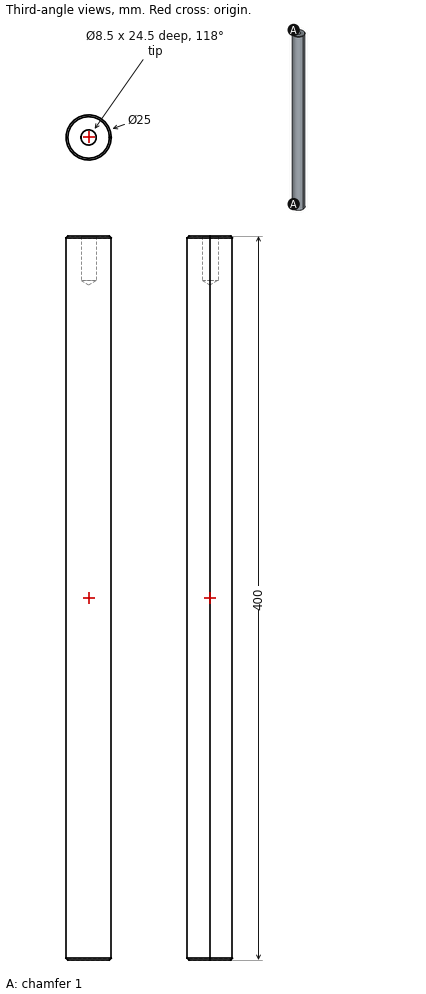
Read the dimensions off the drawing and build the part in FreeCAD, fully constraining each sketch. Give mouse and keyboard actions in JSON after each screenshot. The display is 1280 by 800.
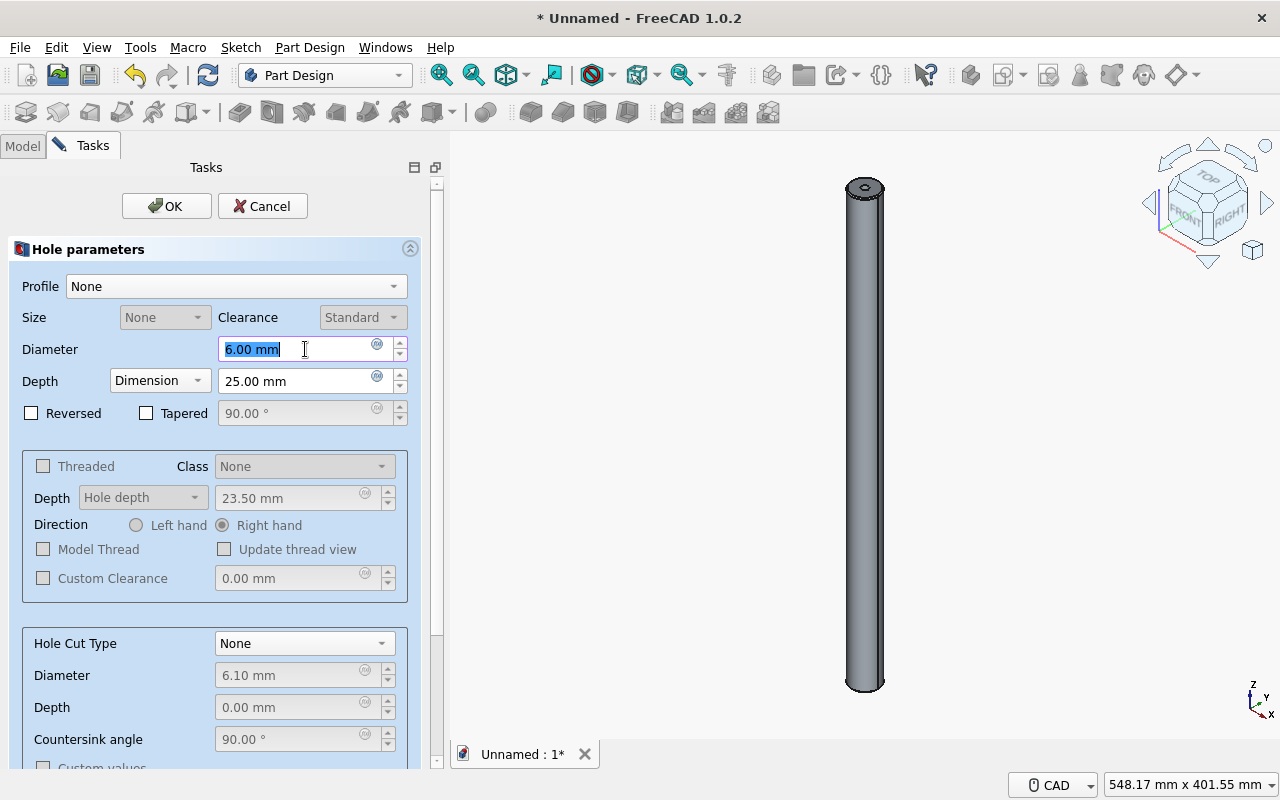
{"action": "type", "text": "8.5"}
{"action": "key", "text": "Tab"}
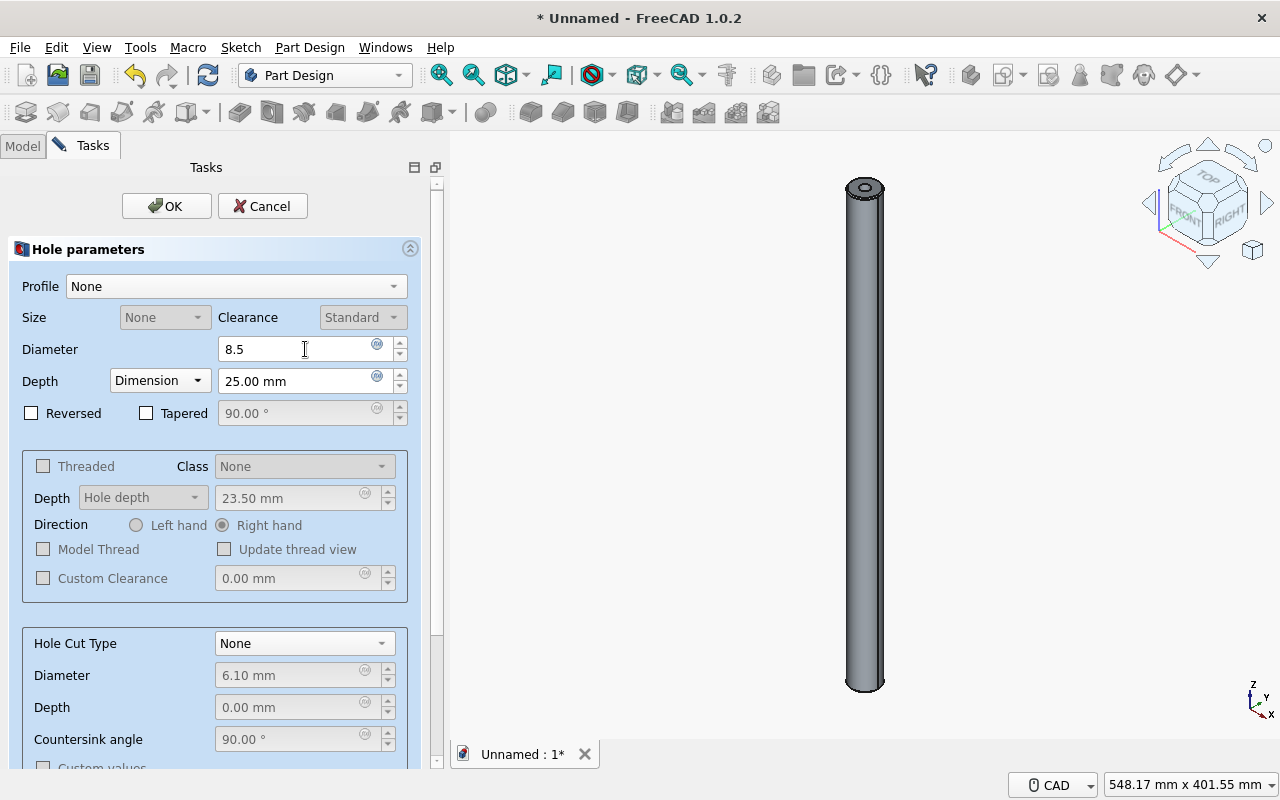
{"action": "triple_click", "coordinate": [305, 381]}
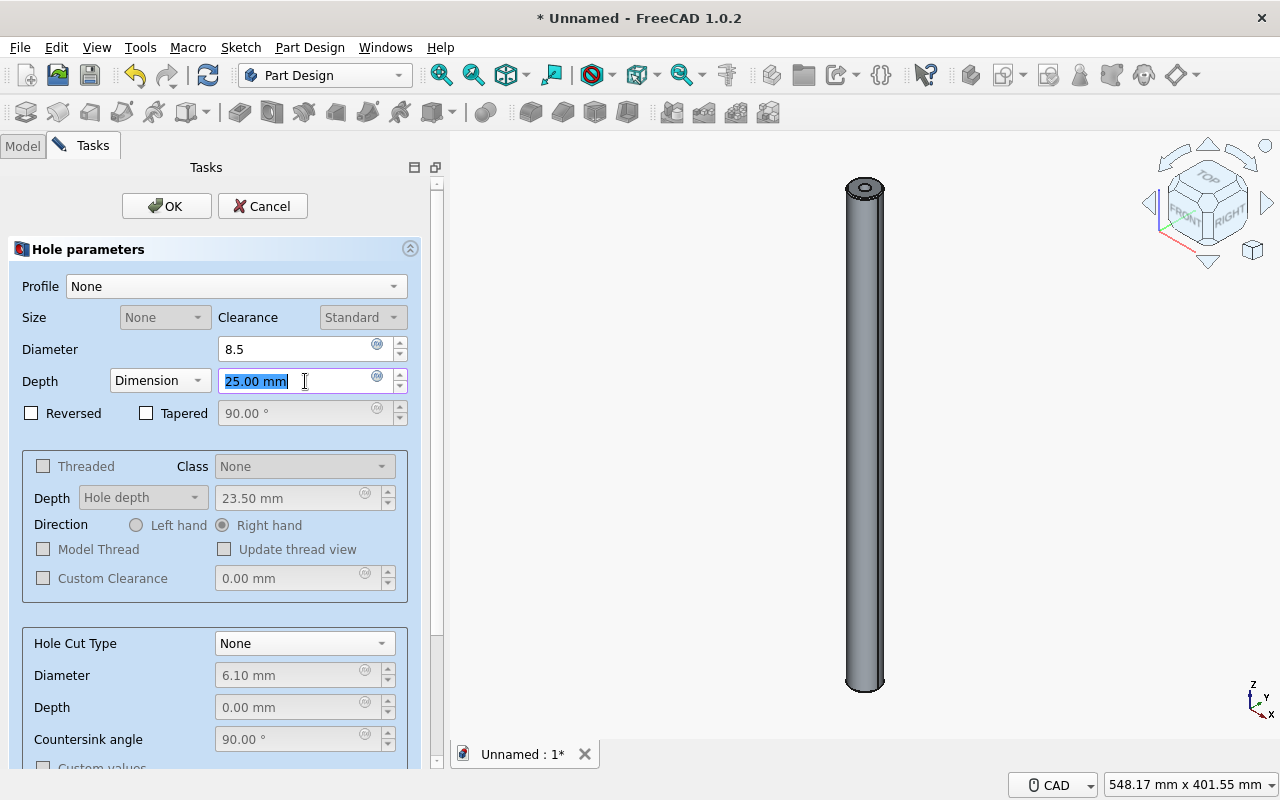
{"action": "type", "text": "24.5"}
{"action": "key", "text": "Tab"}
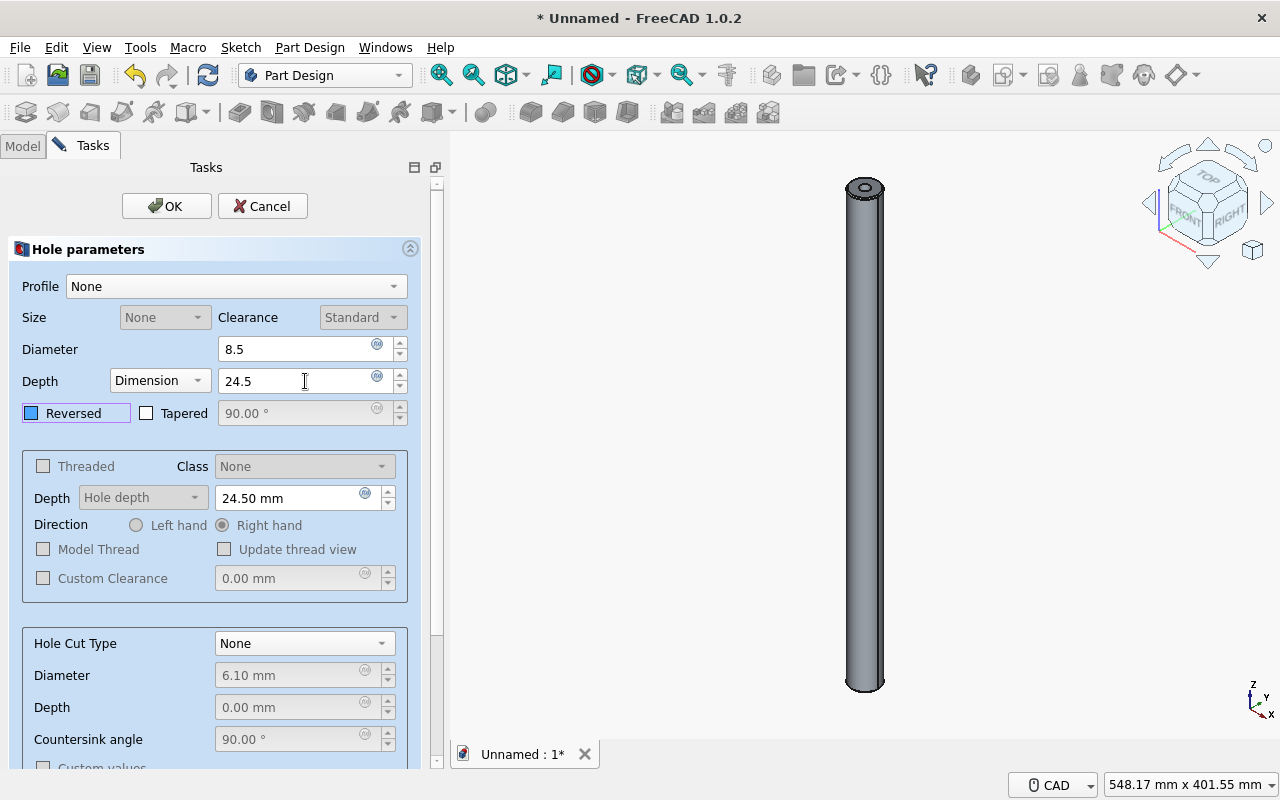
{"action": "left_click", "coordinate": [167, 206]}